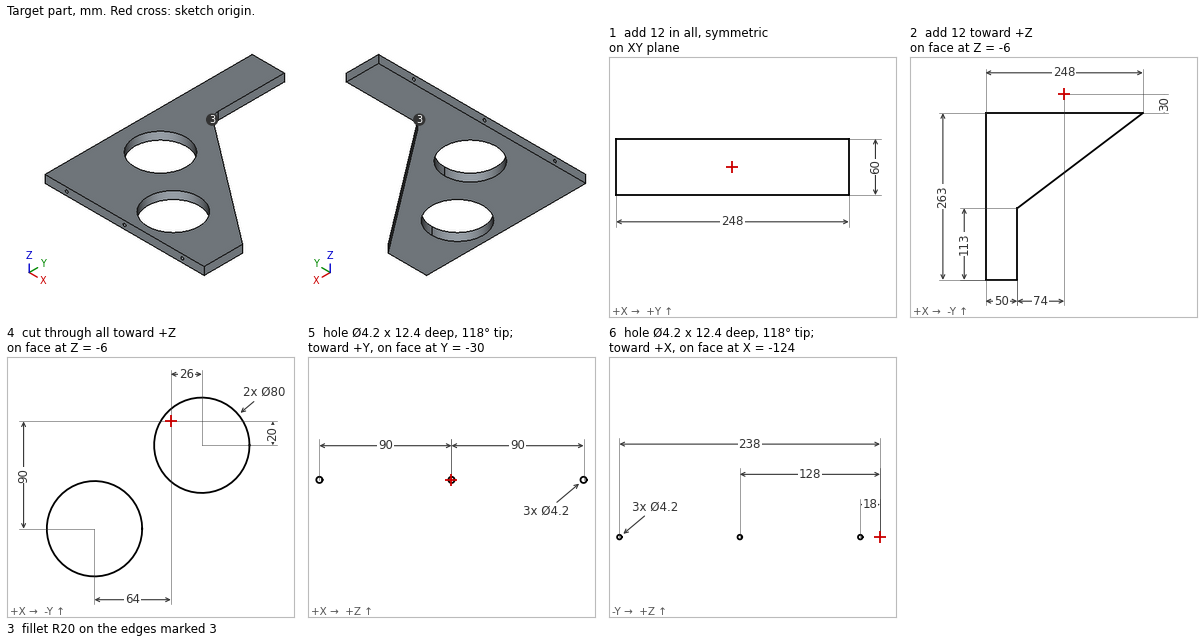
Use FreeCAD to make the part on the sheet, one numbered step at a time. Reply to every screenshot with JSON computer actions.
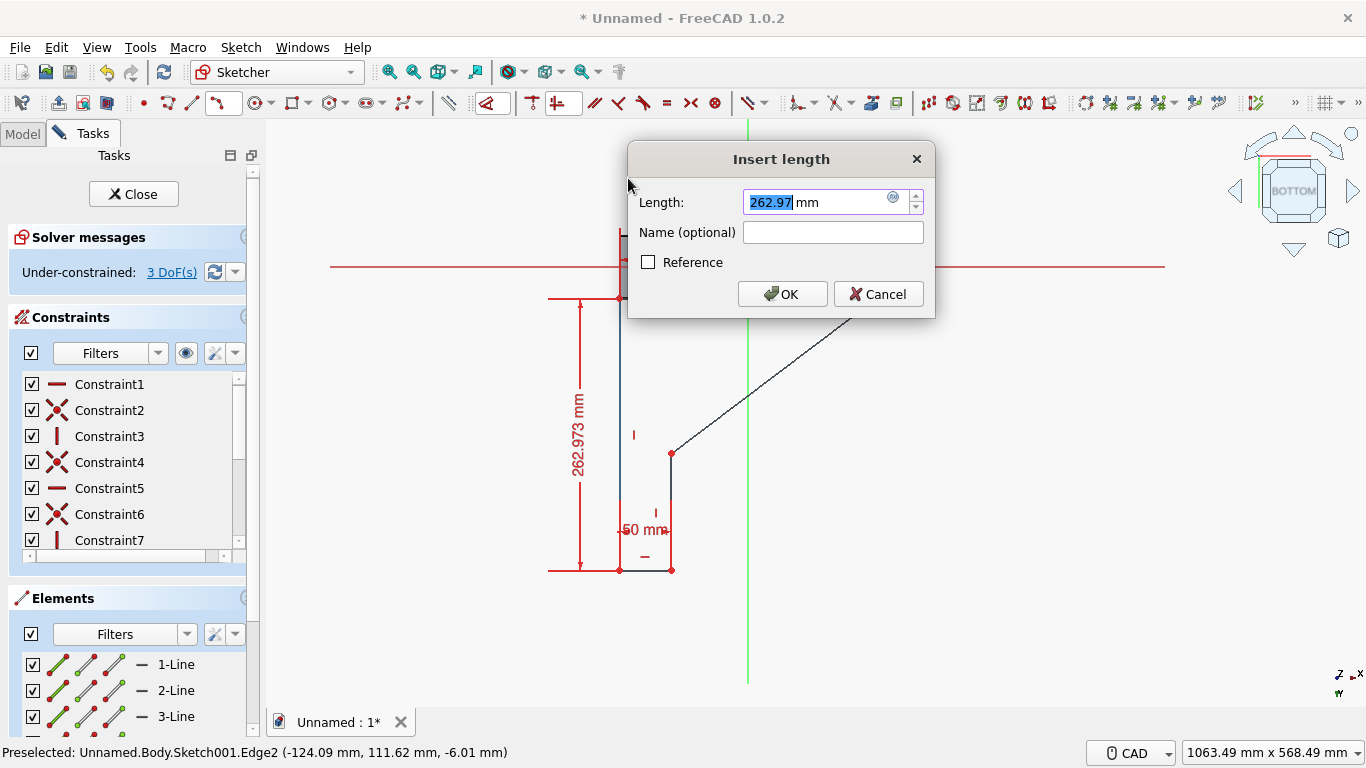
{"action": "type", "text": "263"}
{"action": "key", "text": "Return"}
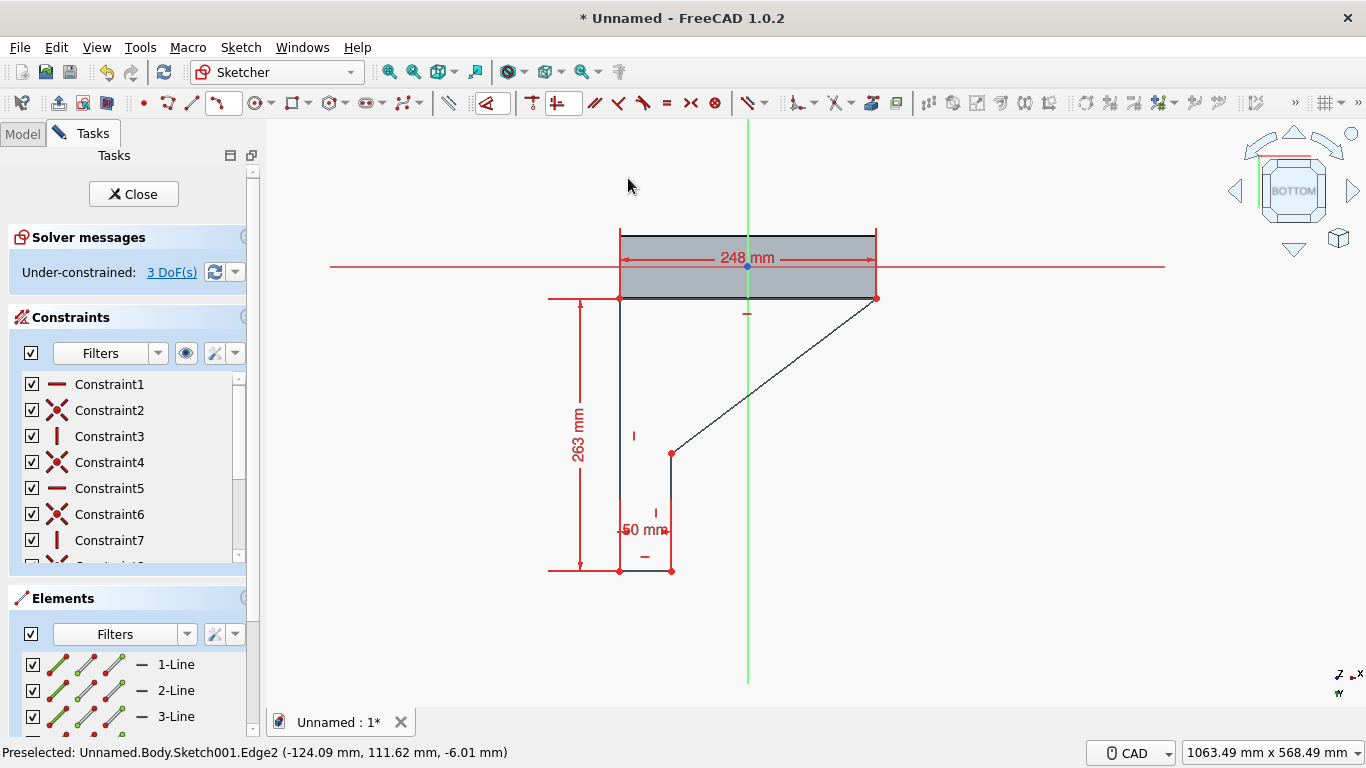
{"action": "left_click", "coordinate": [671, 536]}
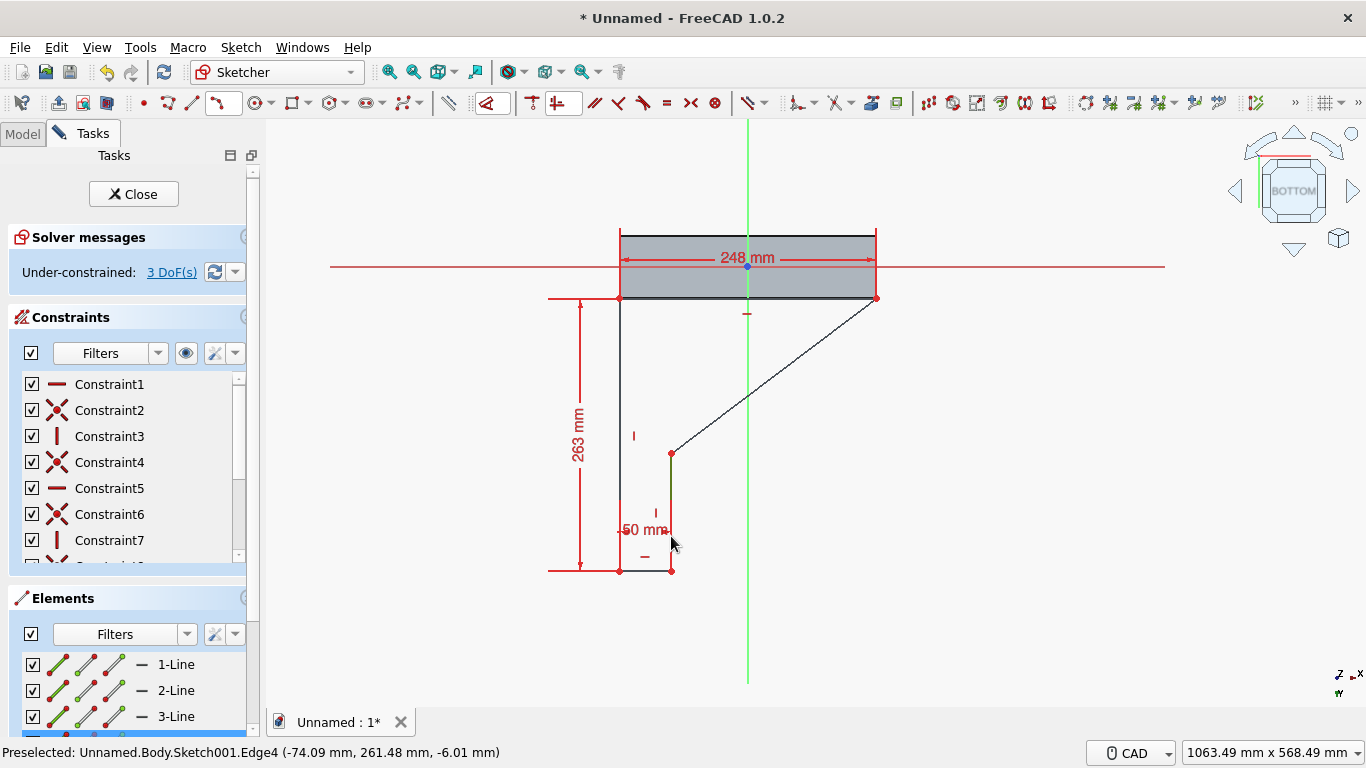
{"action": "left_click", "coordinate": [504, 104]}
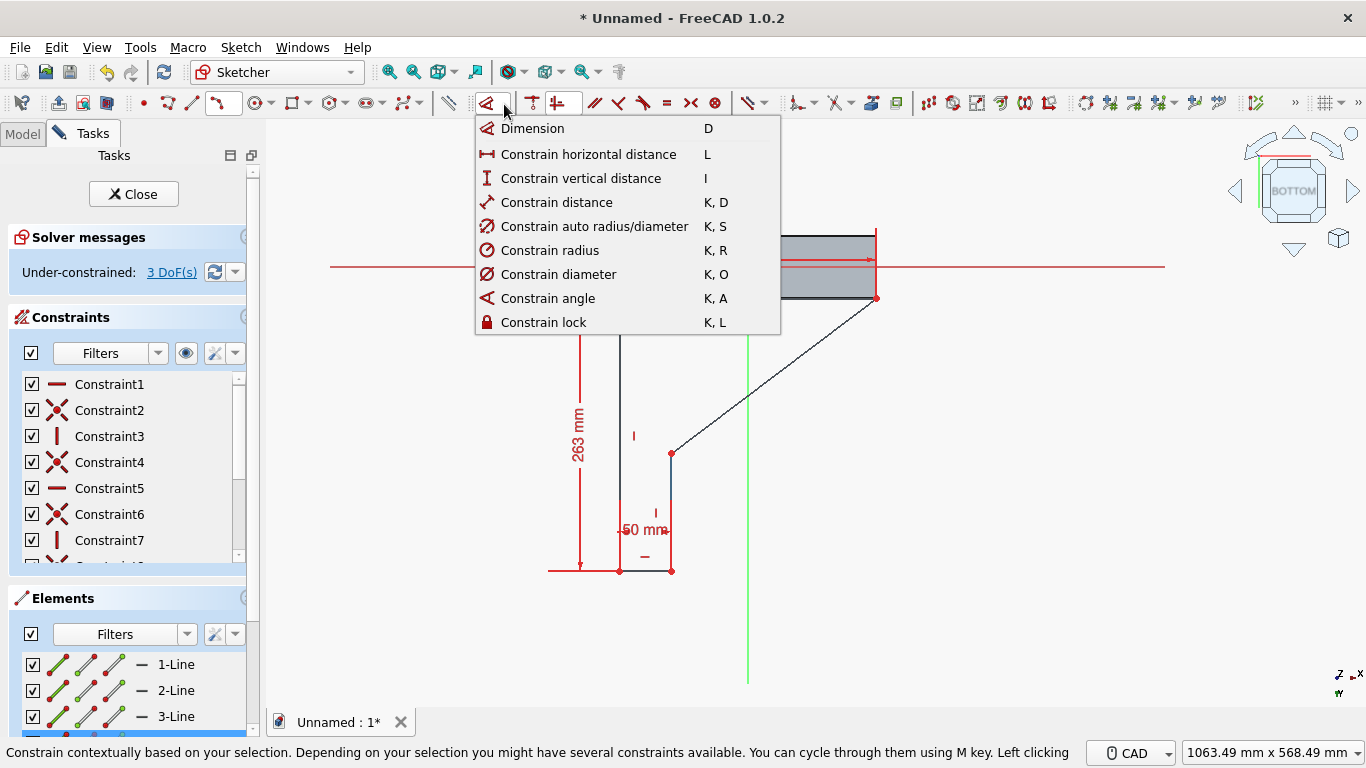
{"action": "left_click", "coordinate": [628, 178]}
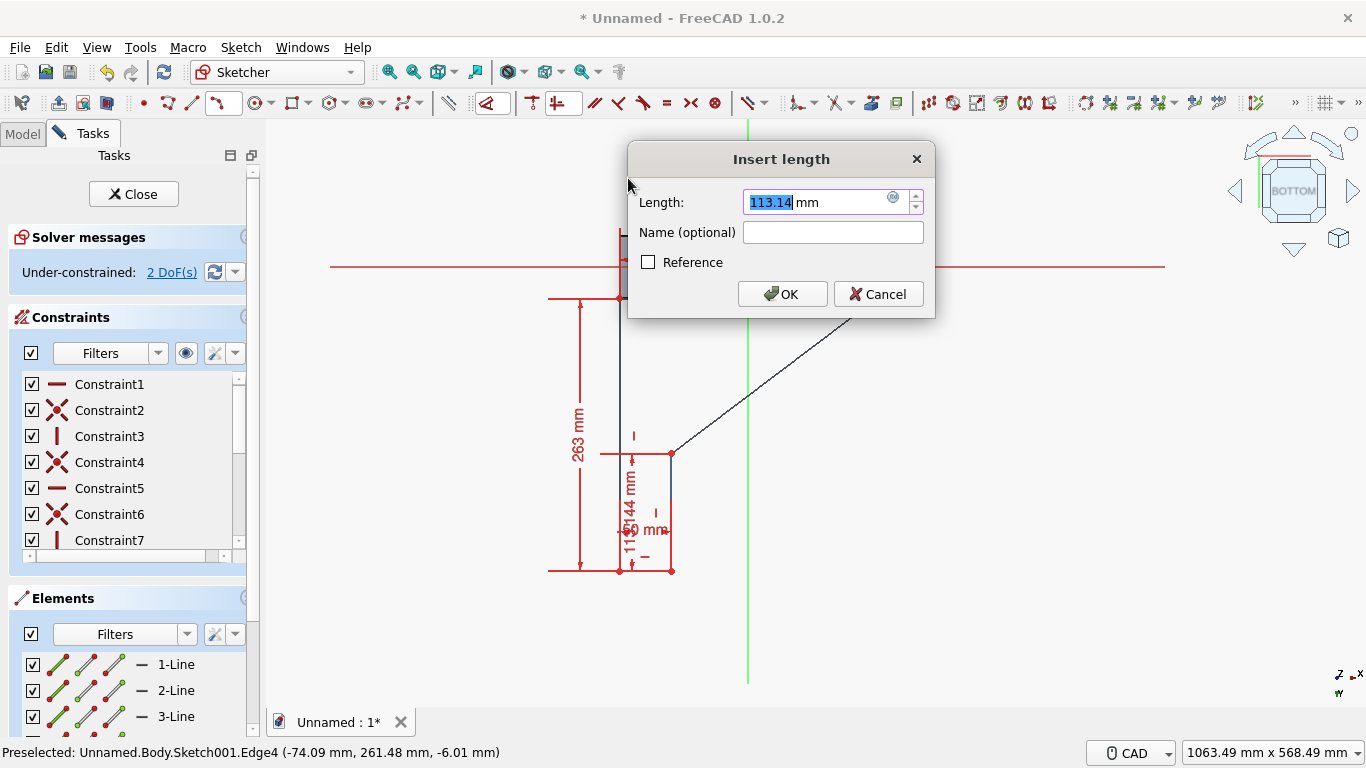
{"action": "type", "text": "113"}
{"action": "key", "text": "Return"}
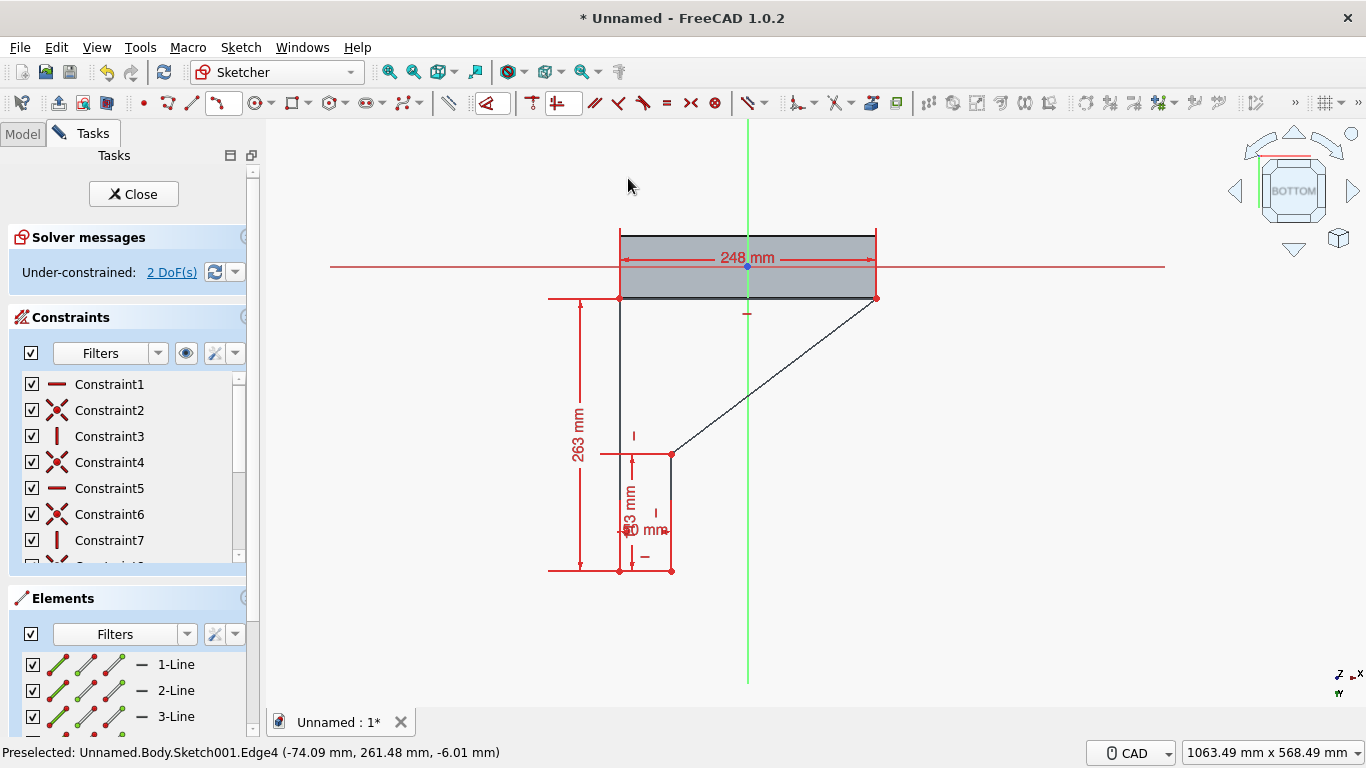
{"action": "scroll", "coordinate": [876, 299], "scroll_direction": "up", "scroll_amount": 2}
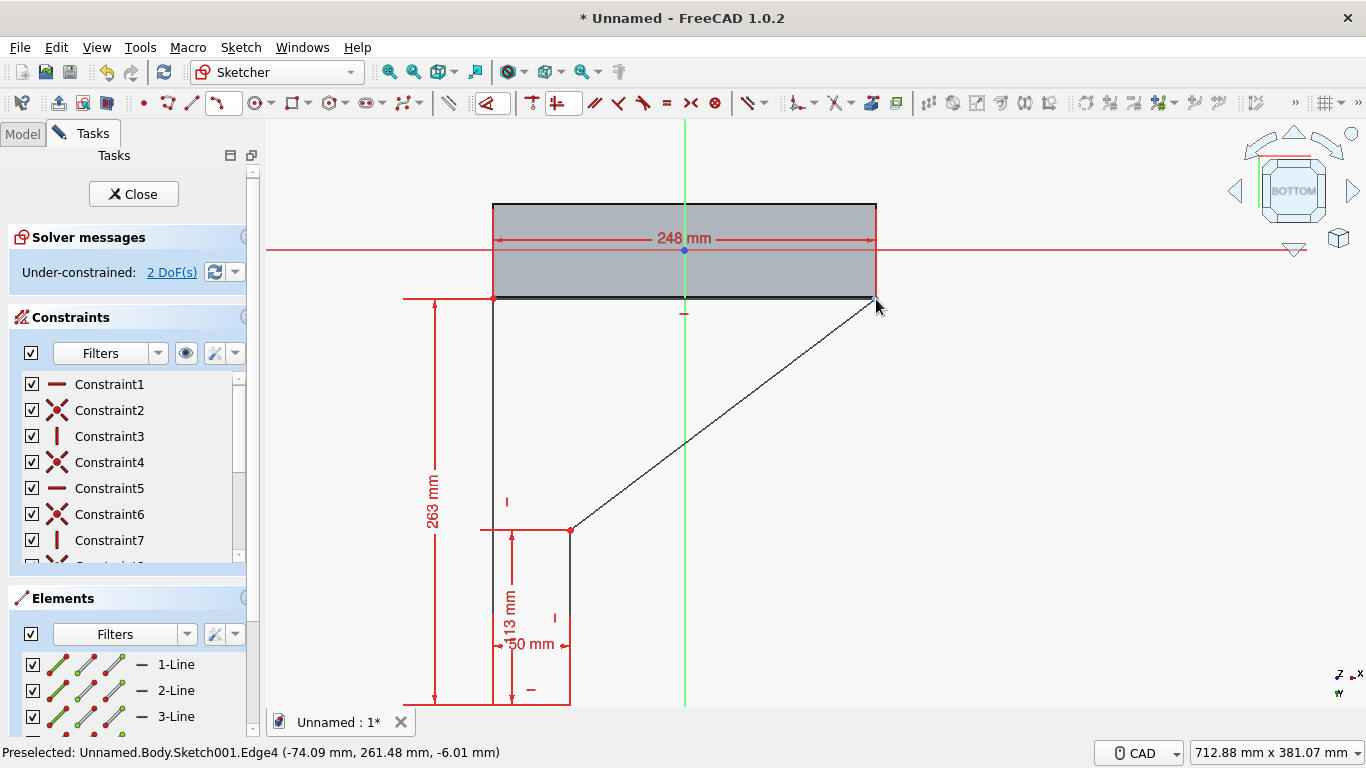
{"action": "left_click", "coordinate": [876, 299]}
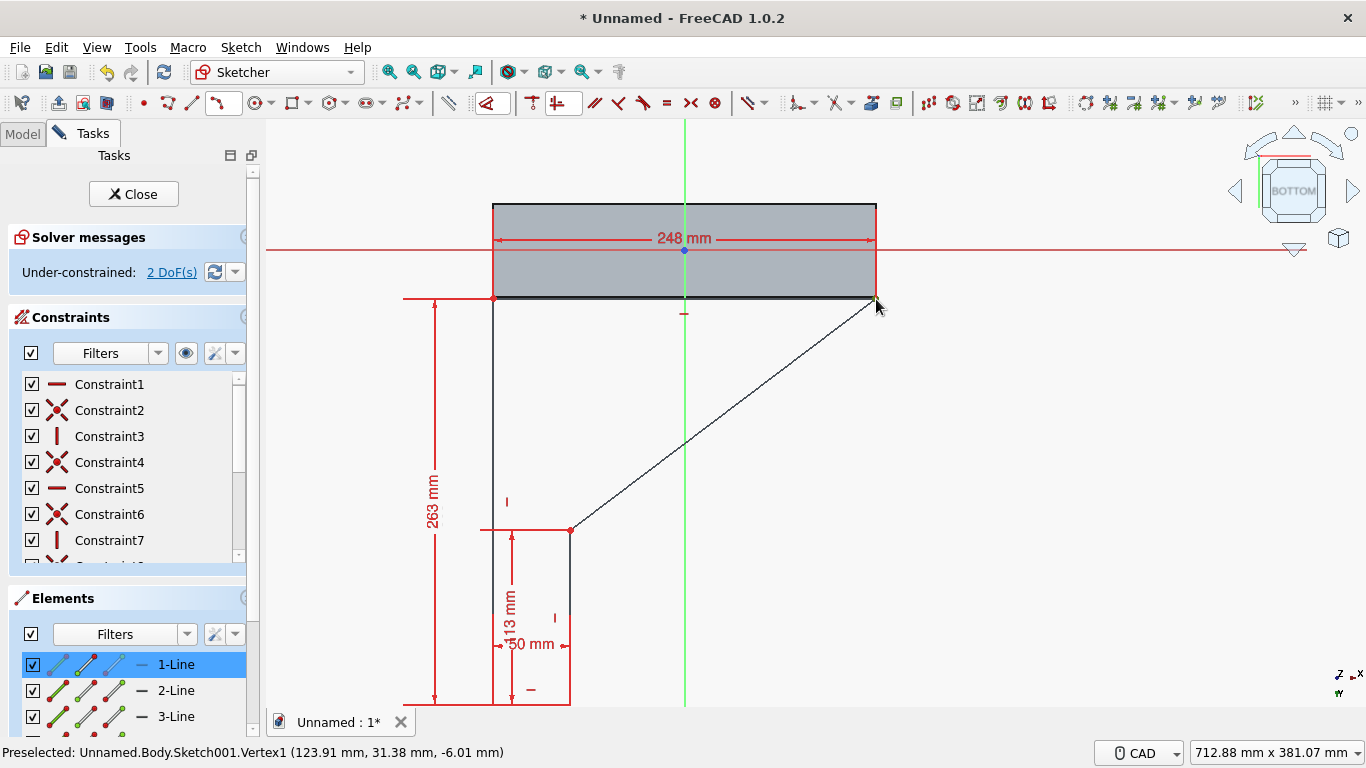
{"action": "key", "text": "i"}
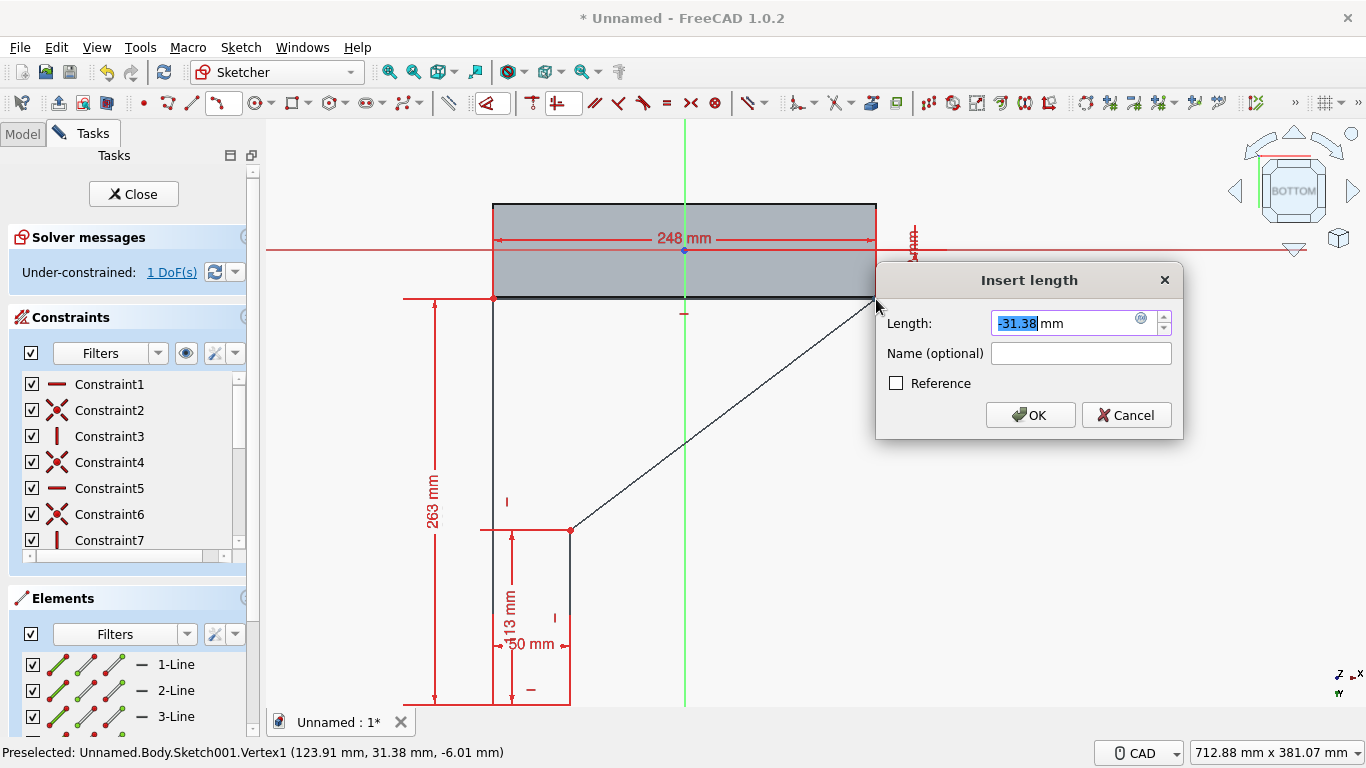
{"action": "type", "text": "-30"}
{"action": "key", "text": "Return"}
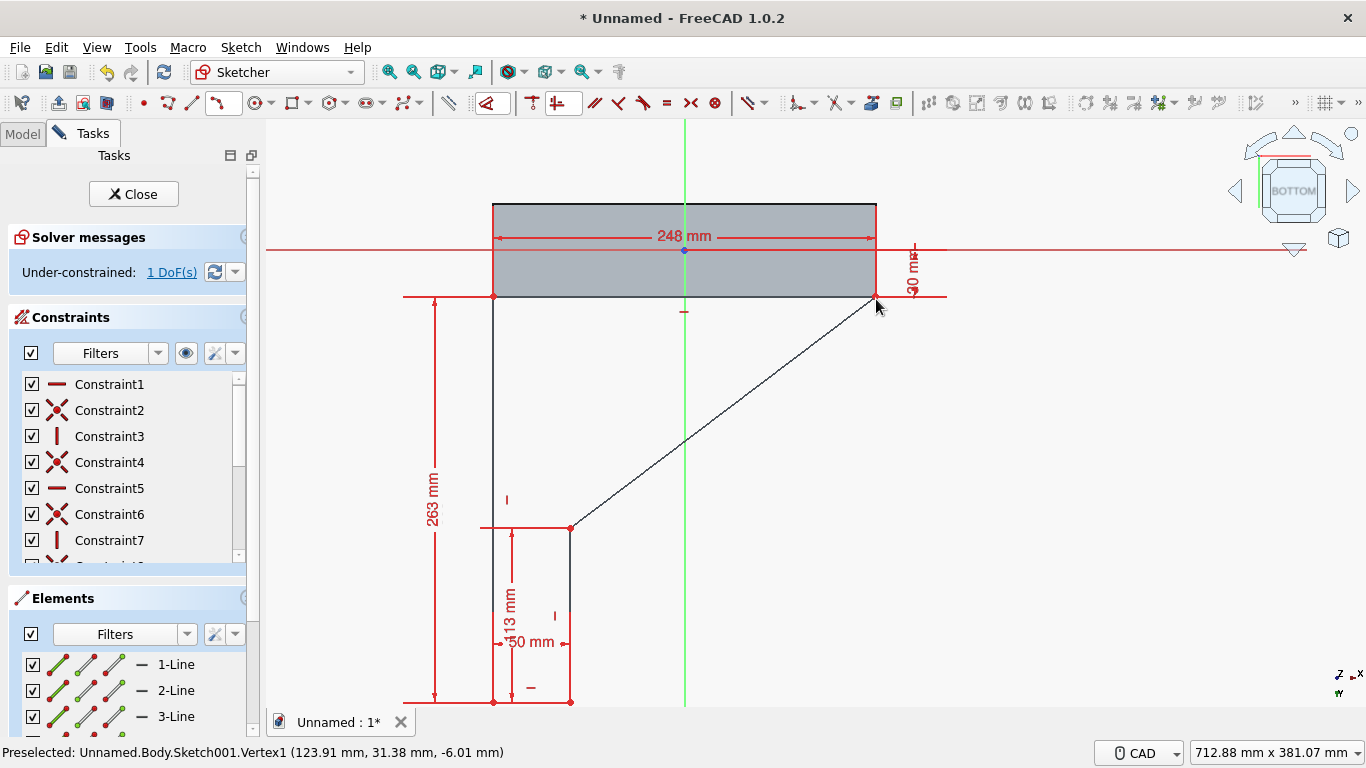
{"action": "scroll", "coordinate": [1031, 147], "scroll_direction": "down", "scroll_amount": 1}